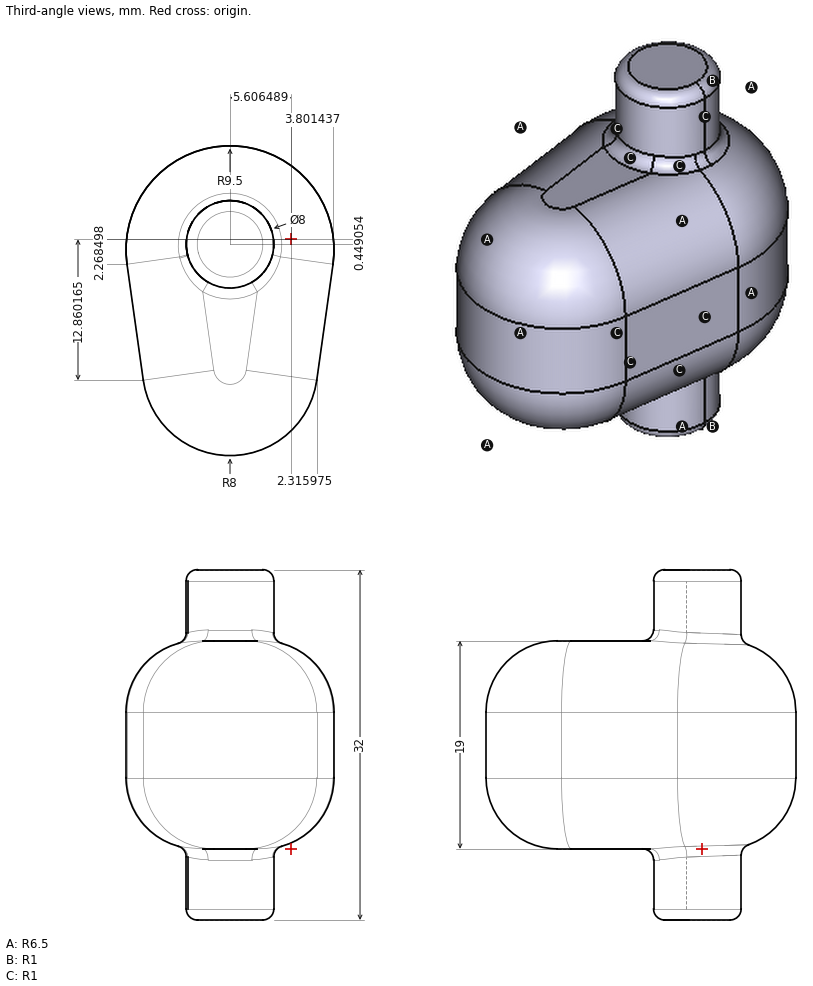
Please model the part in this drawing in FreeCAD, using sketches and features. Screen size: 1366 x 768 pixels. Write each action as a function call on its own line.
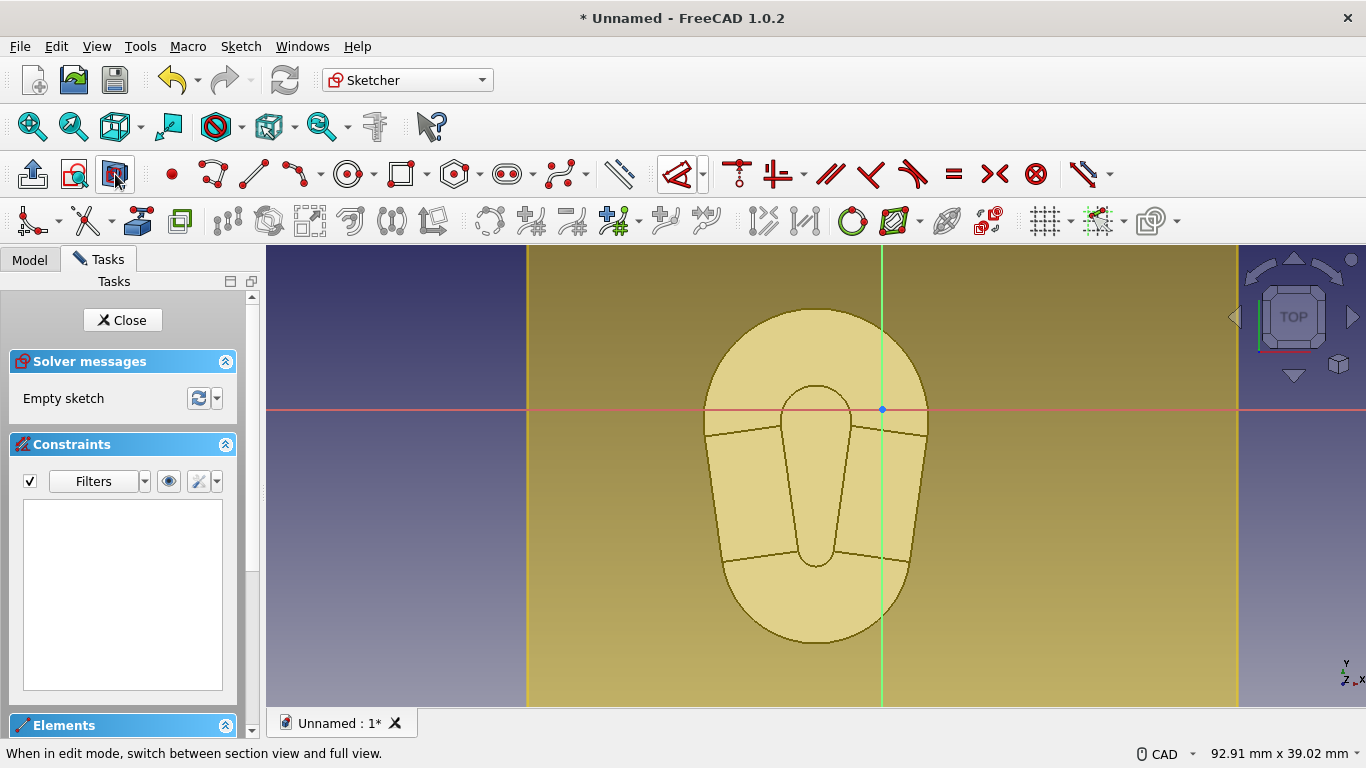
scroll(859, 389, up, 6)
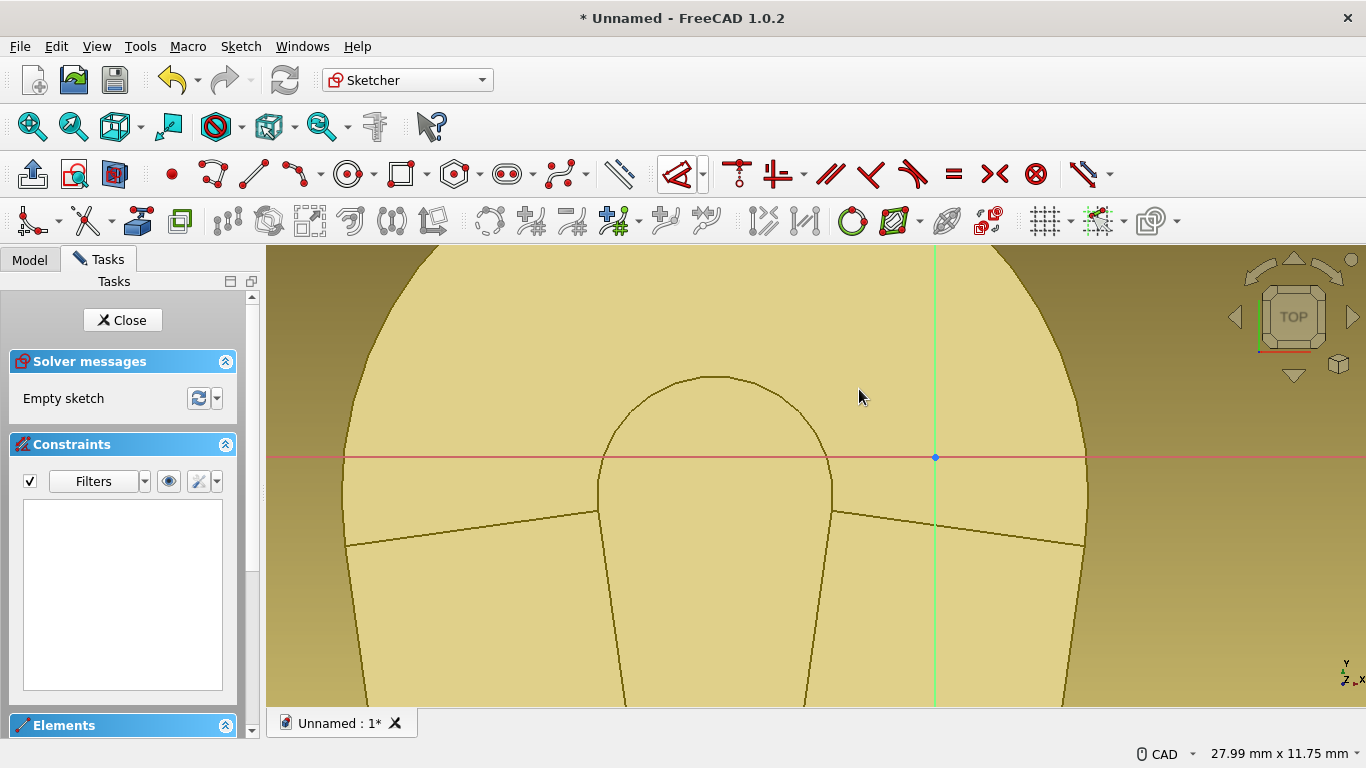
key(g)
key(c)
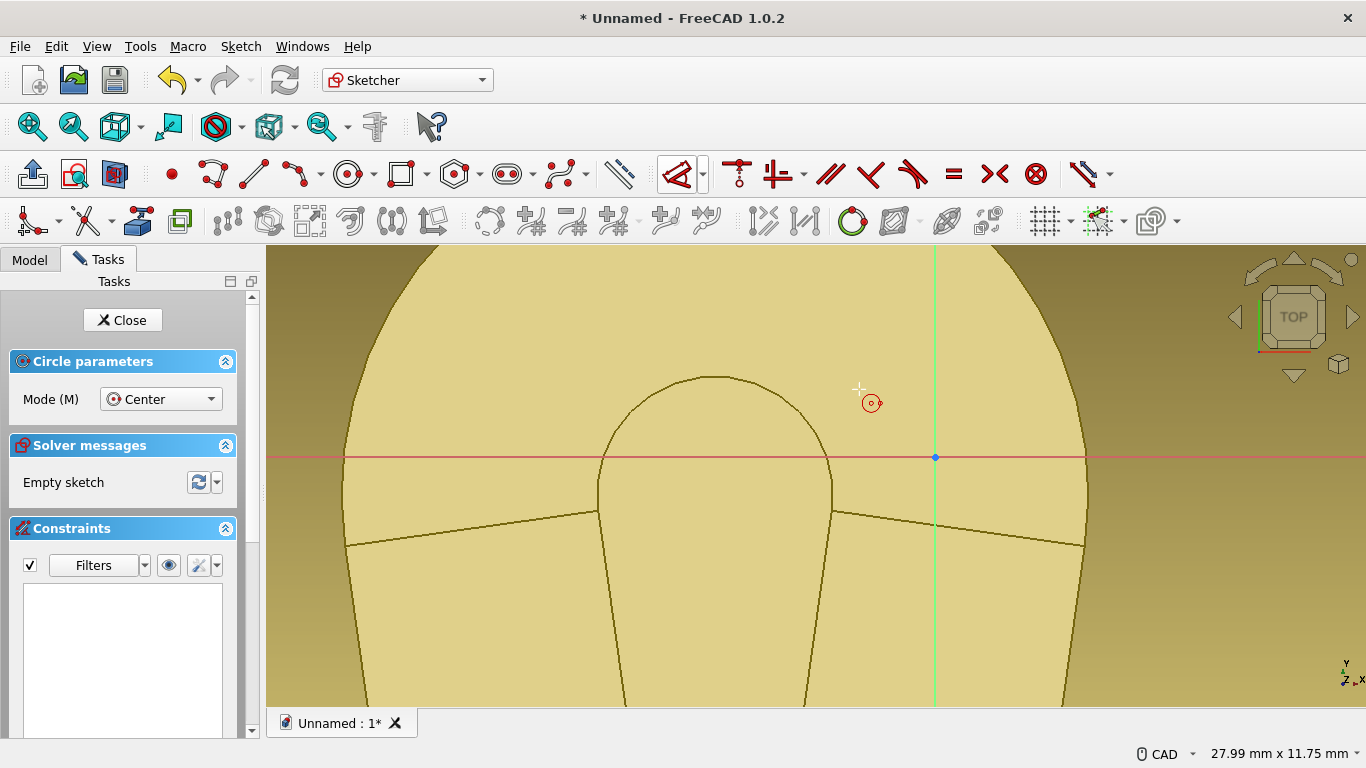
click(715, 475)
move(826, 364)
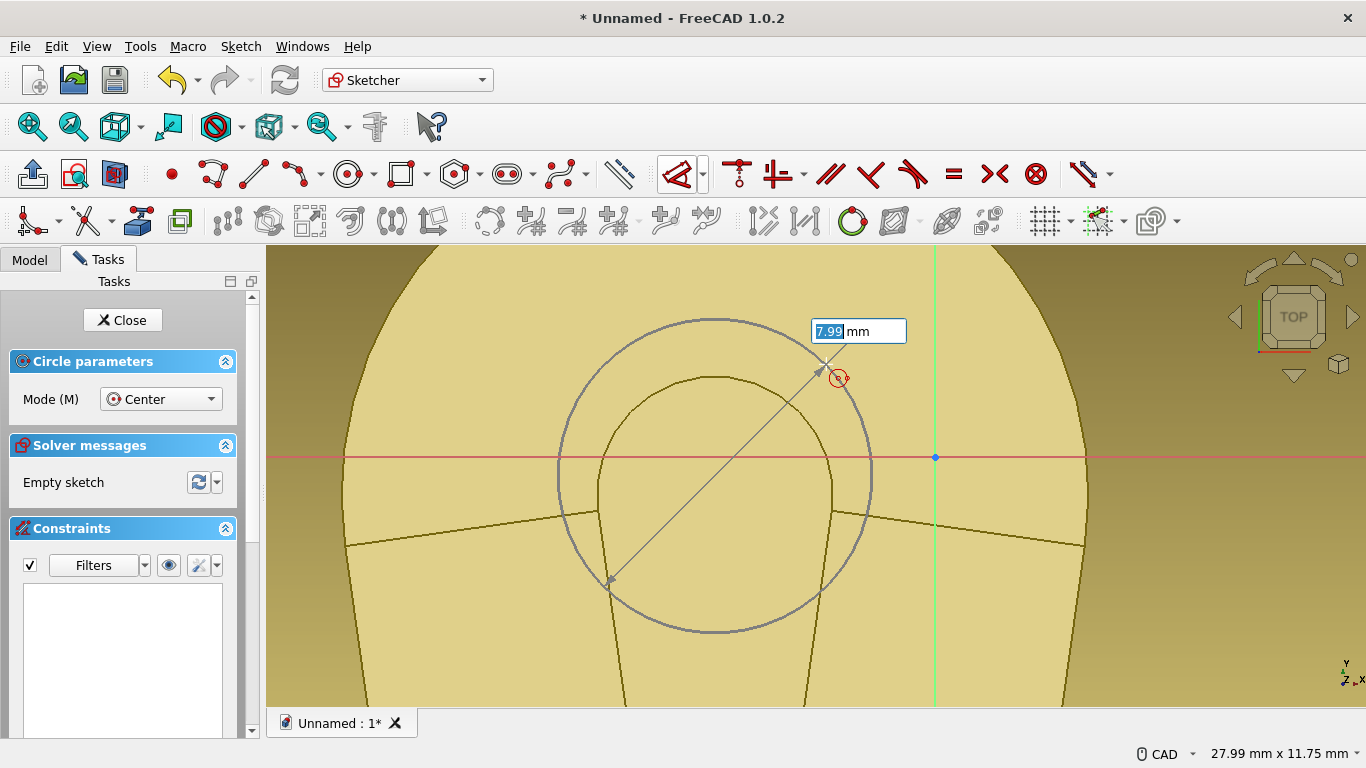
text(8)
key(Return)
key(Escape)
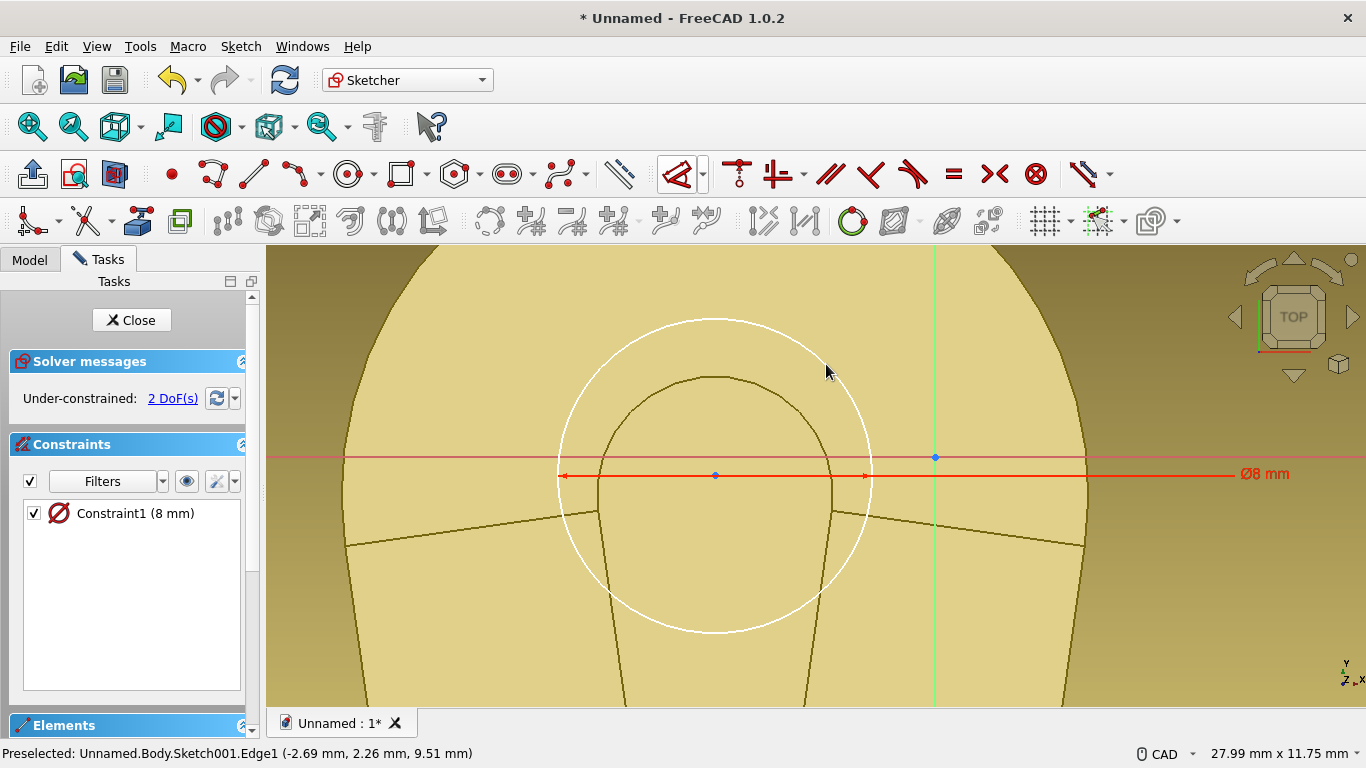
click(715, 476)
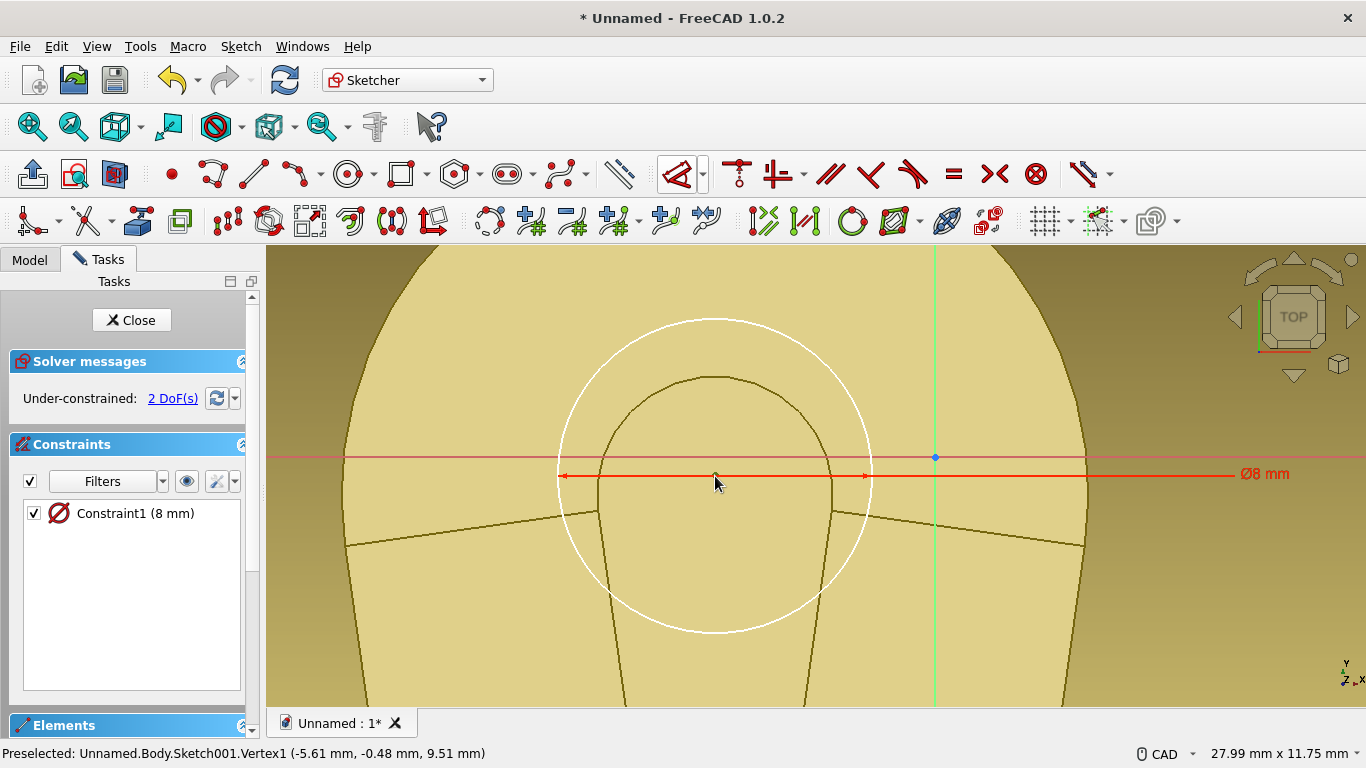
key(l)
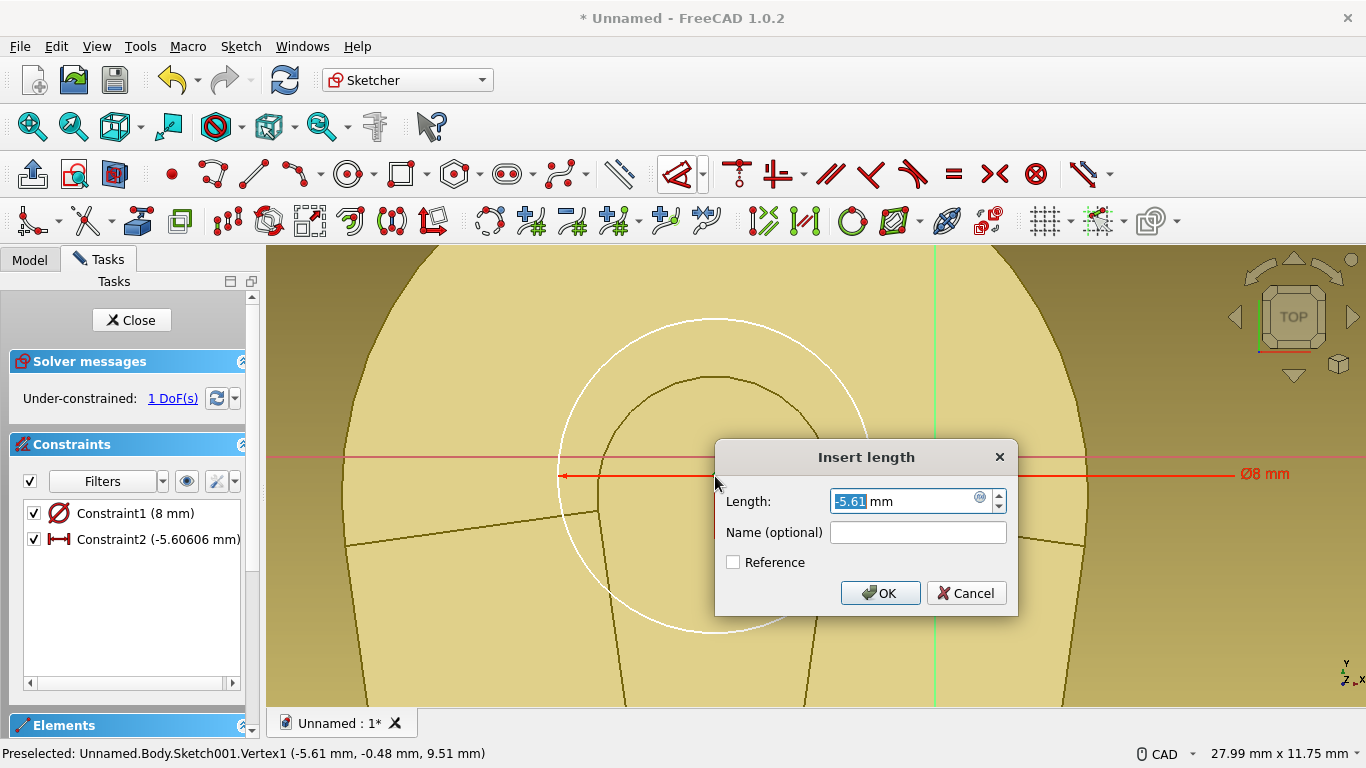
text(-5.606489)
key(Return)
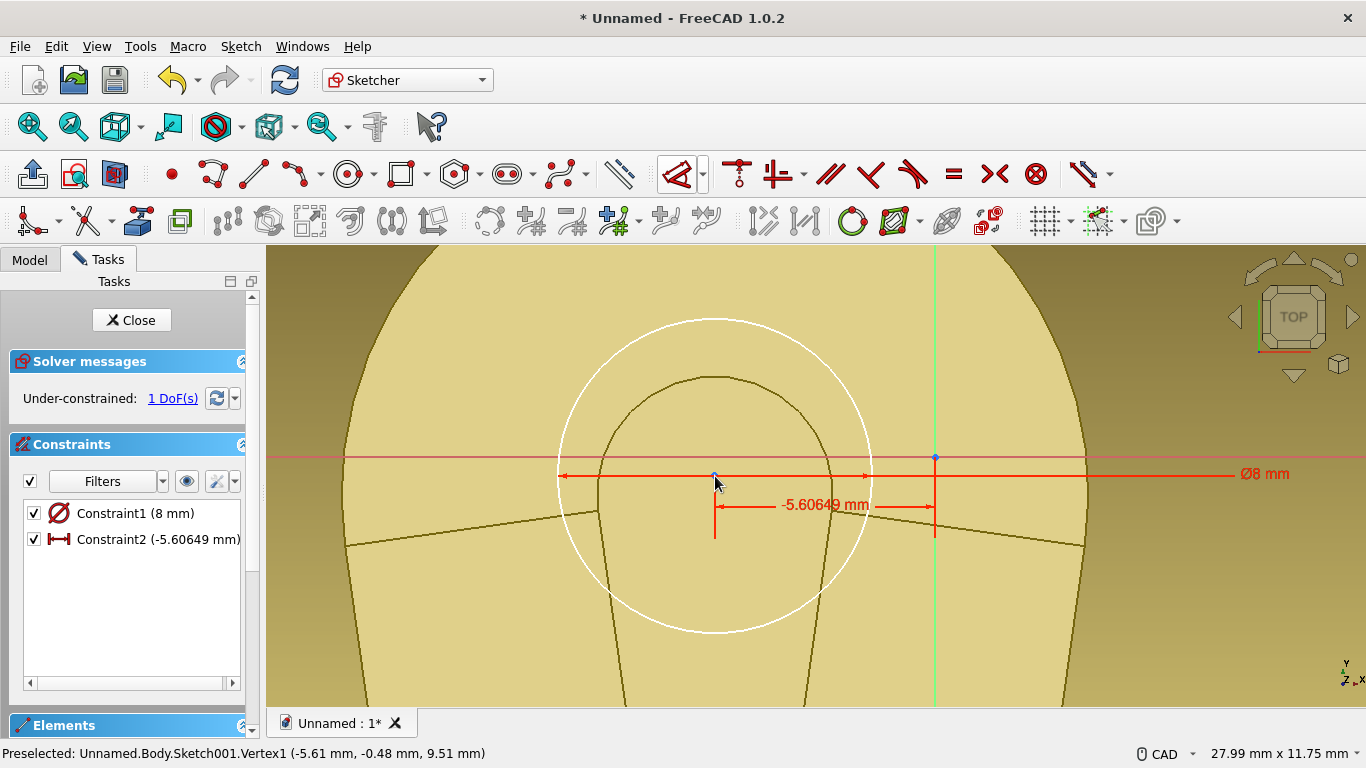
scroll(715, 476, up, 5)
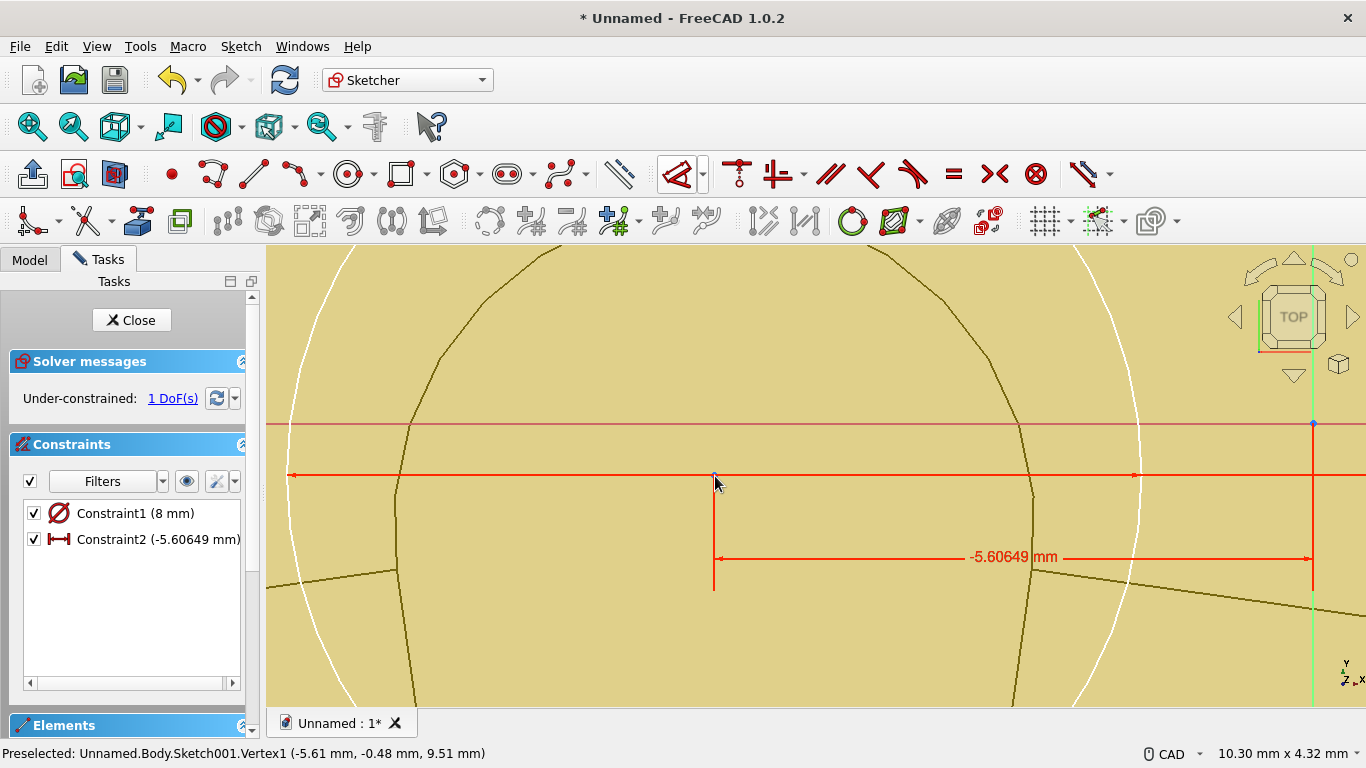
click(714, 475)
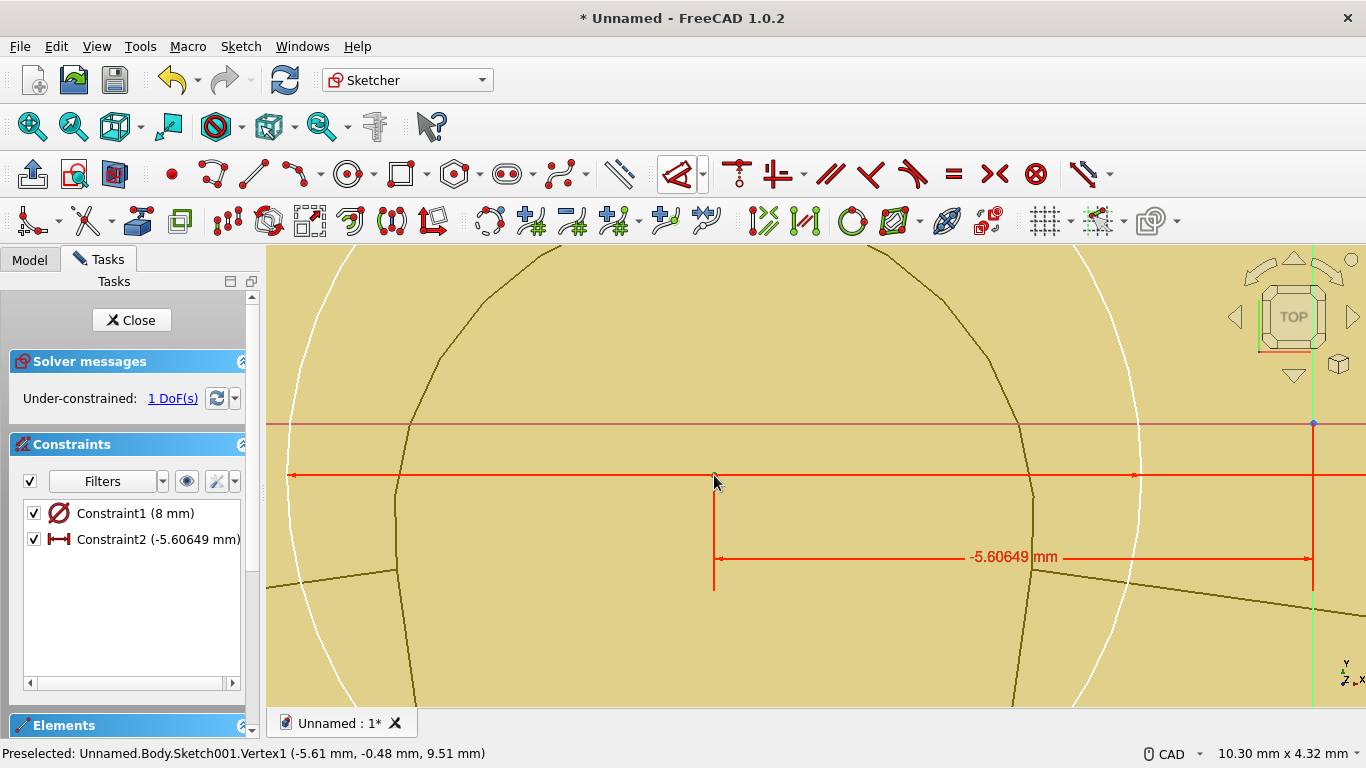
key(i)